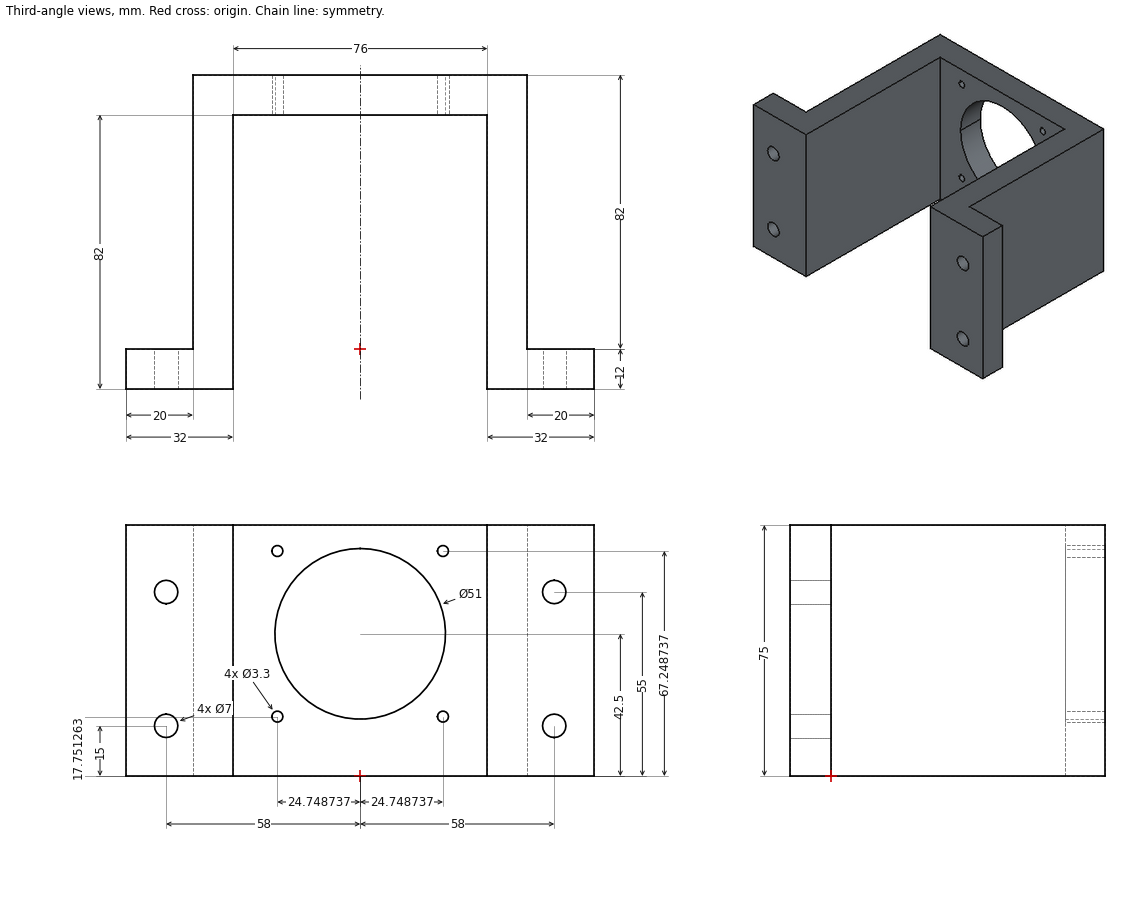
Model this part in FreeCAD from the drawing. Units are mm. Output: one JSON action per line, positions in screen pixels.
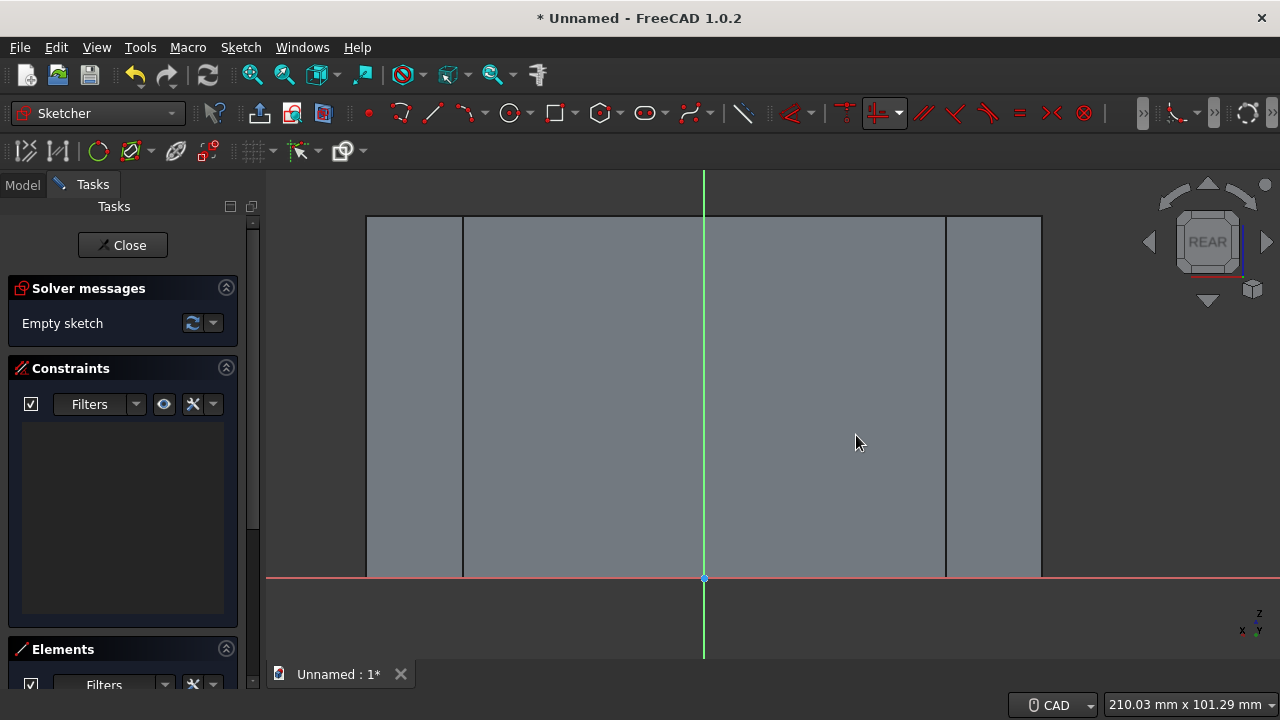
{"action": "left_click", "coordinate": [510, 114]}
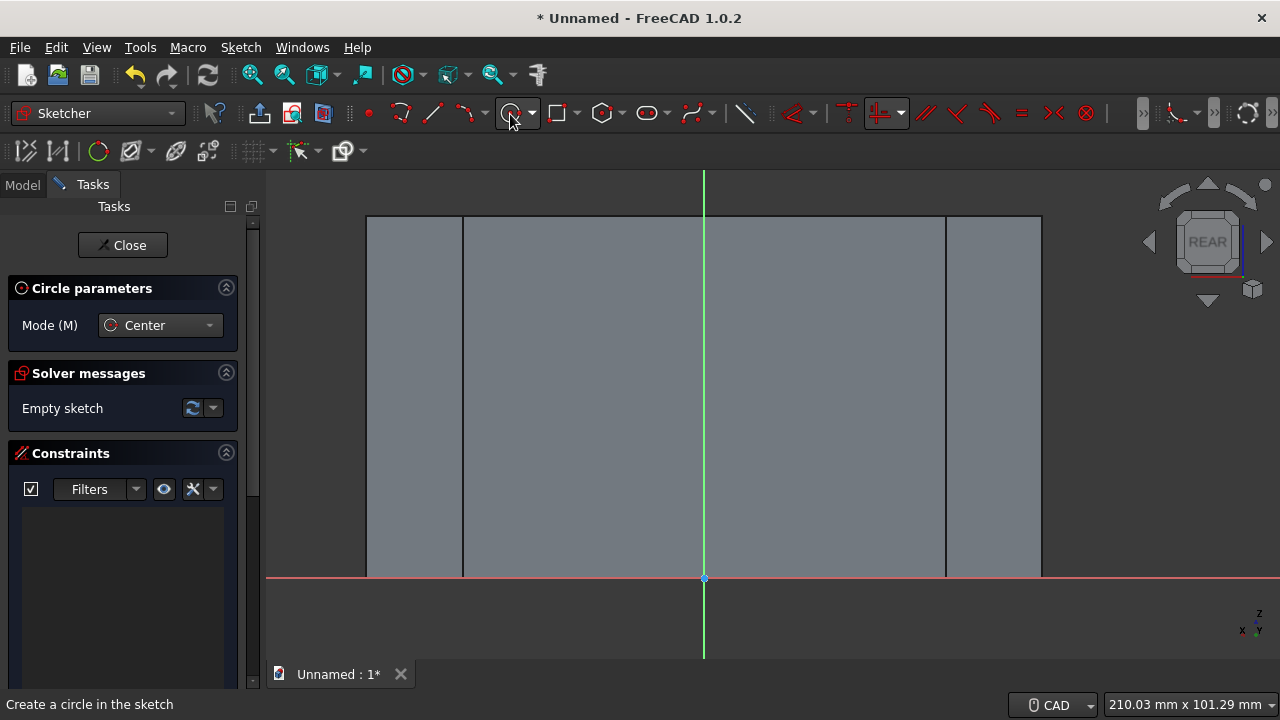
{"action": "left_click", "coordinate": [704, 373]}
{"action": "mouse_move", "coordinate": [791, 286]}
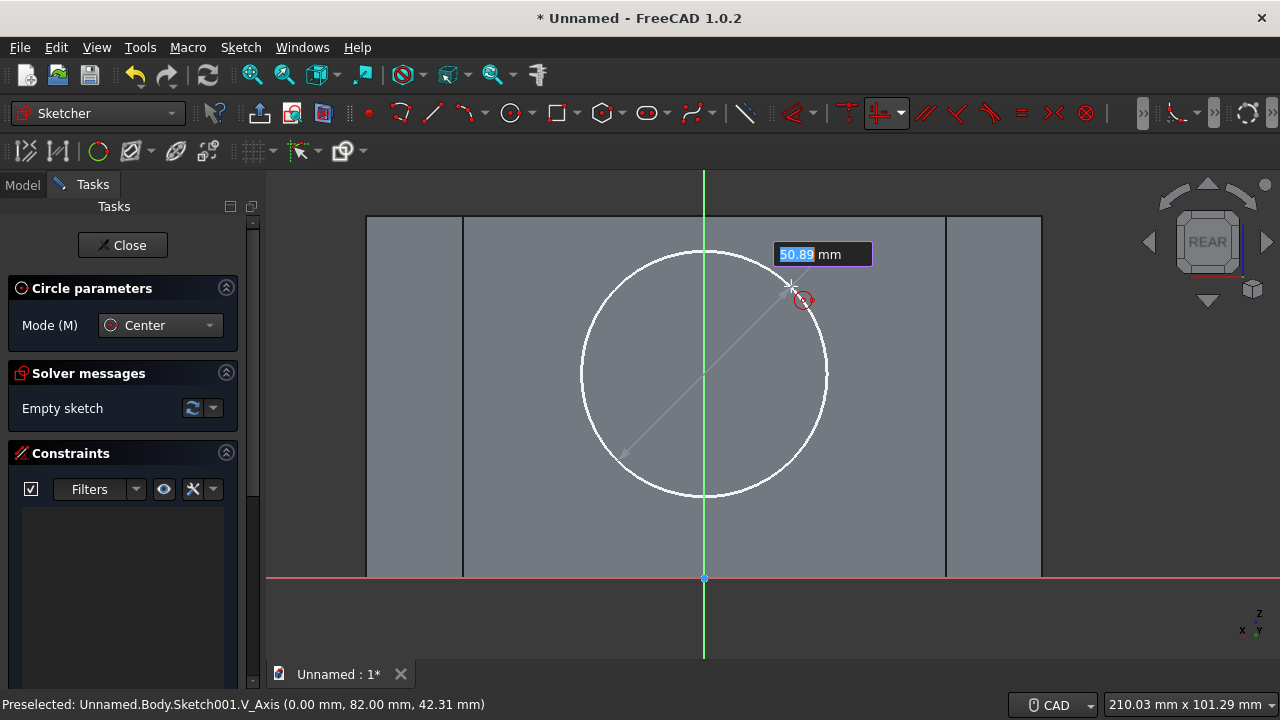
{"action": "type", "text": "51"}
{"action": "key", "text": "Return"}
{"action": "key", "text": "Escape"}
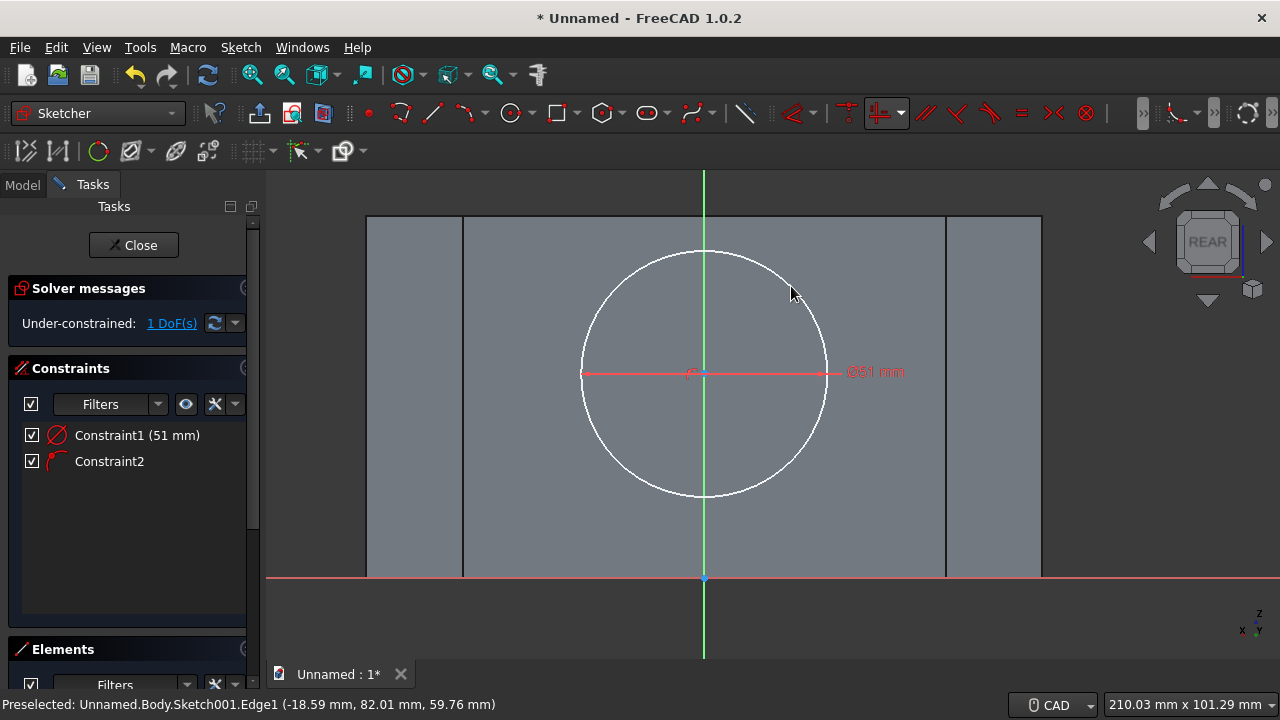
{"action": "left_click", "coordinate": [792, 114]}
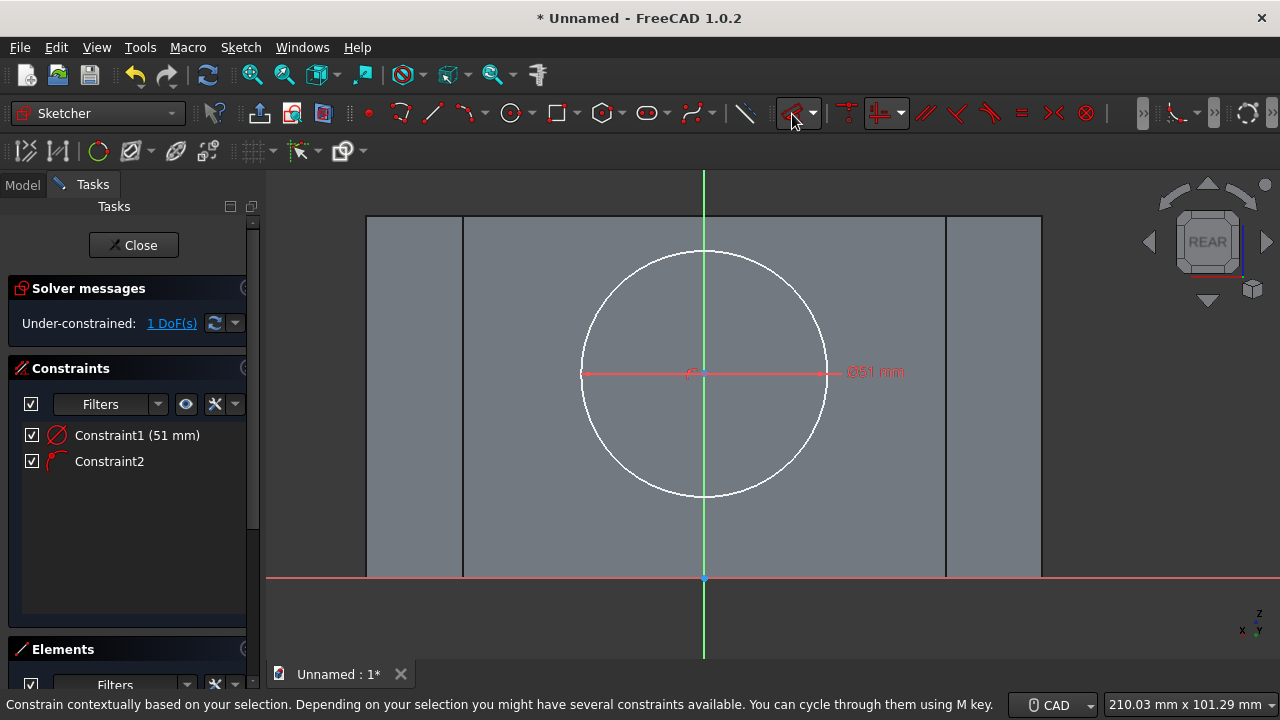
{"action": "left_click", "coordinate": [704, 374]}
{"action": "left_click", "coordinate": [738, 476]}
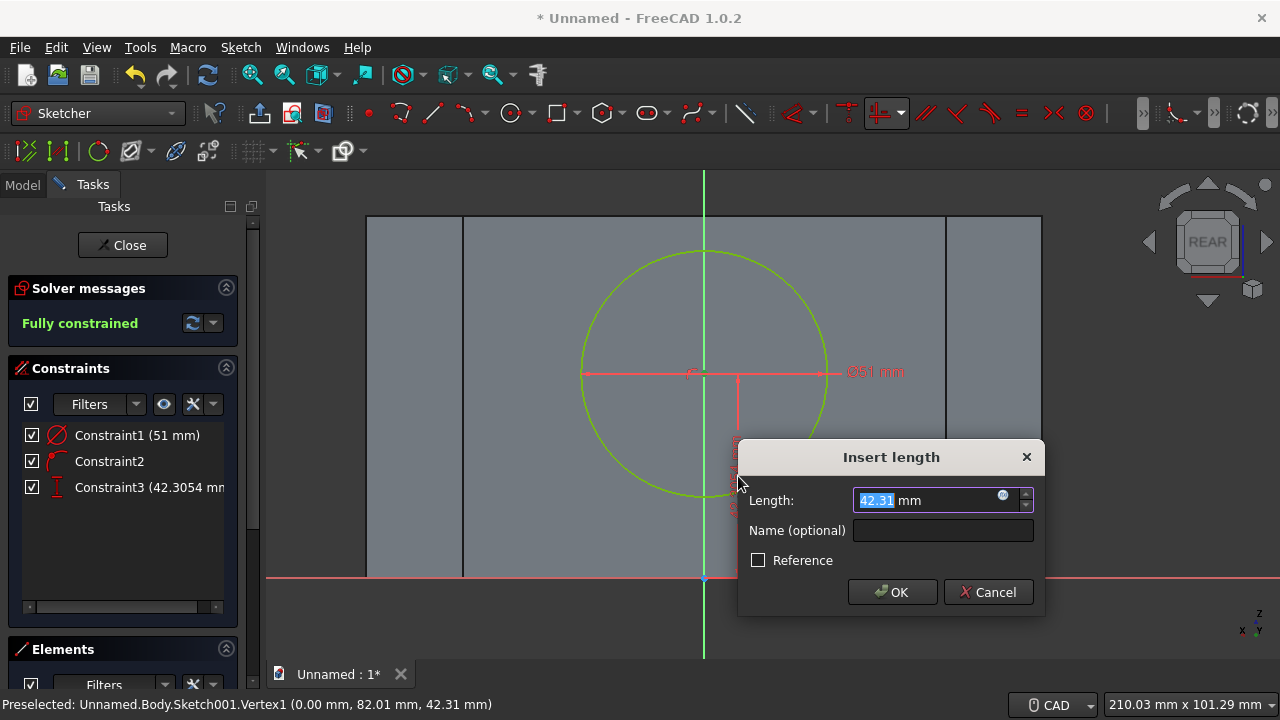
{"action": "type", "text": "42.5"}
{"action": "key", "text": "Return"}
{"action": "key", "text": "Escape"}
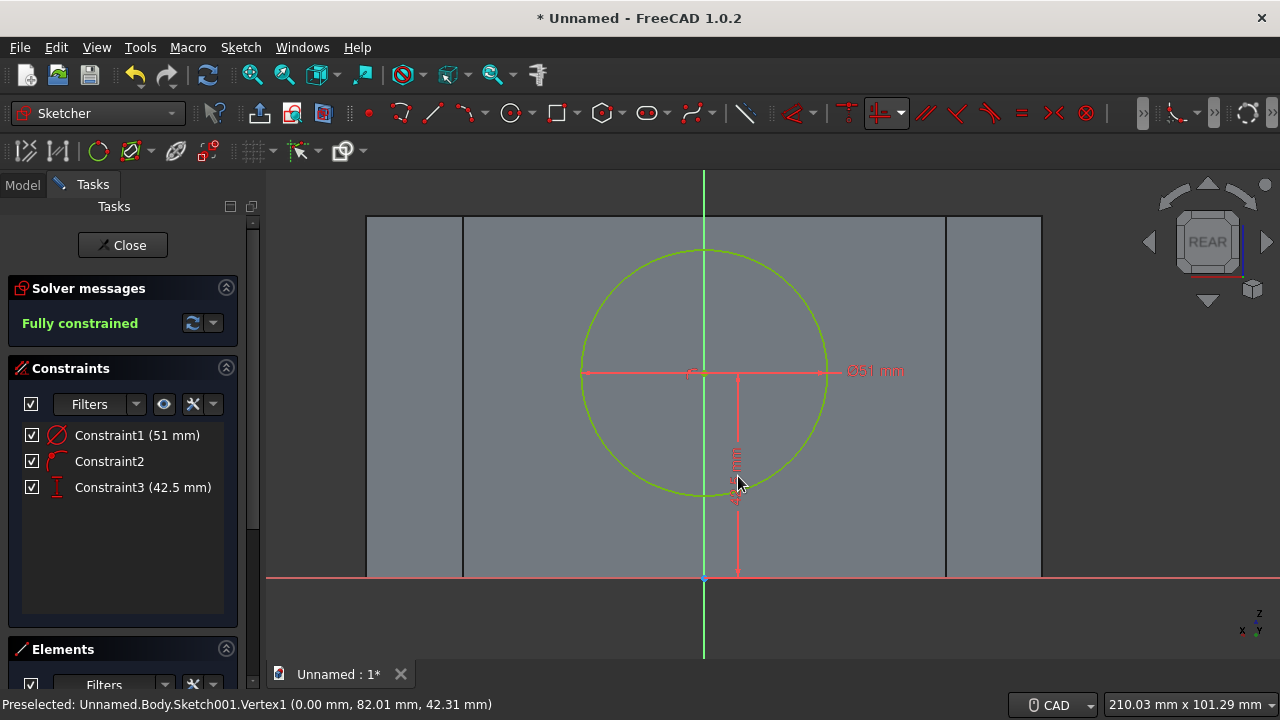
{"action": "left_click", "coordinate": [123, 245]}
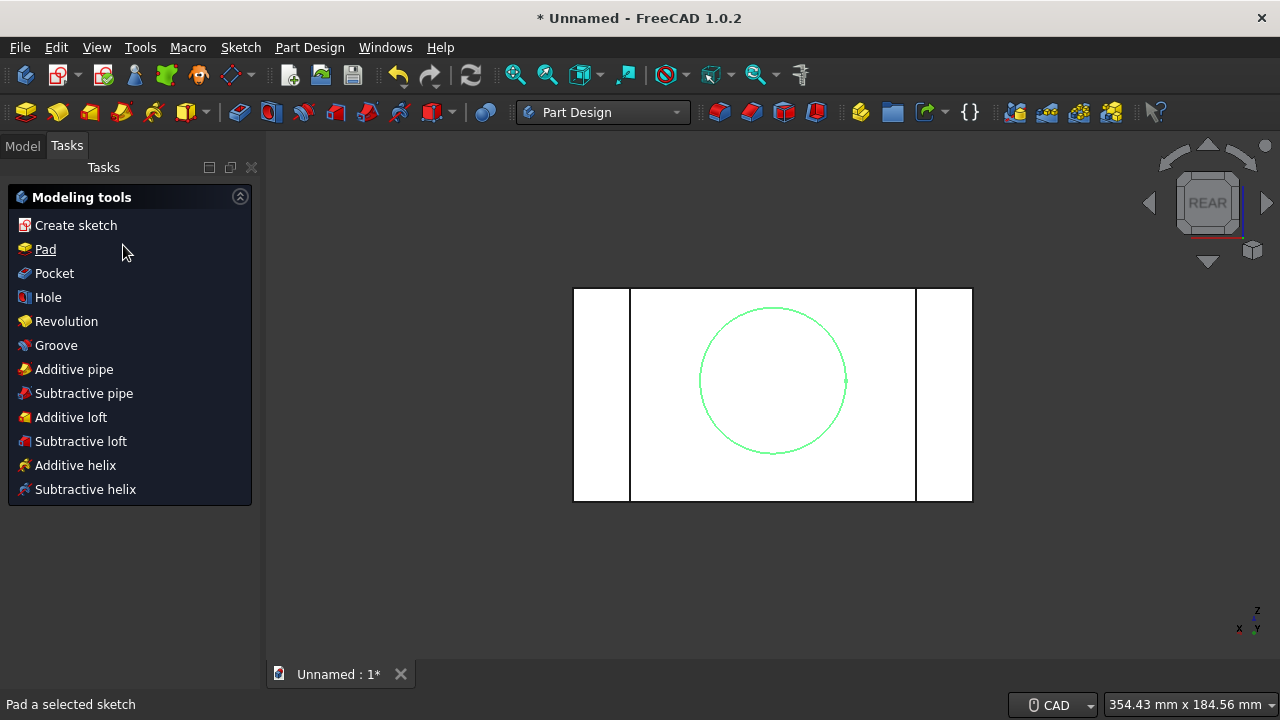
{"action": "left_click", "coordinate": [240, 112]}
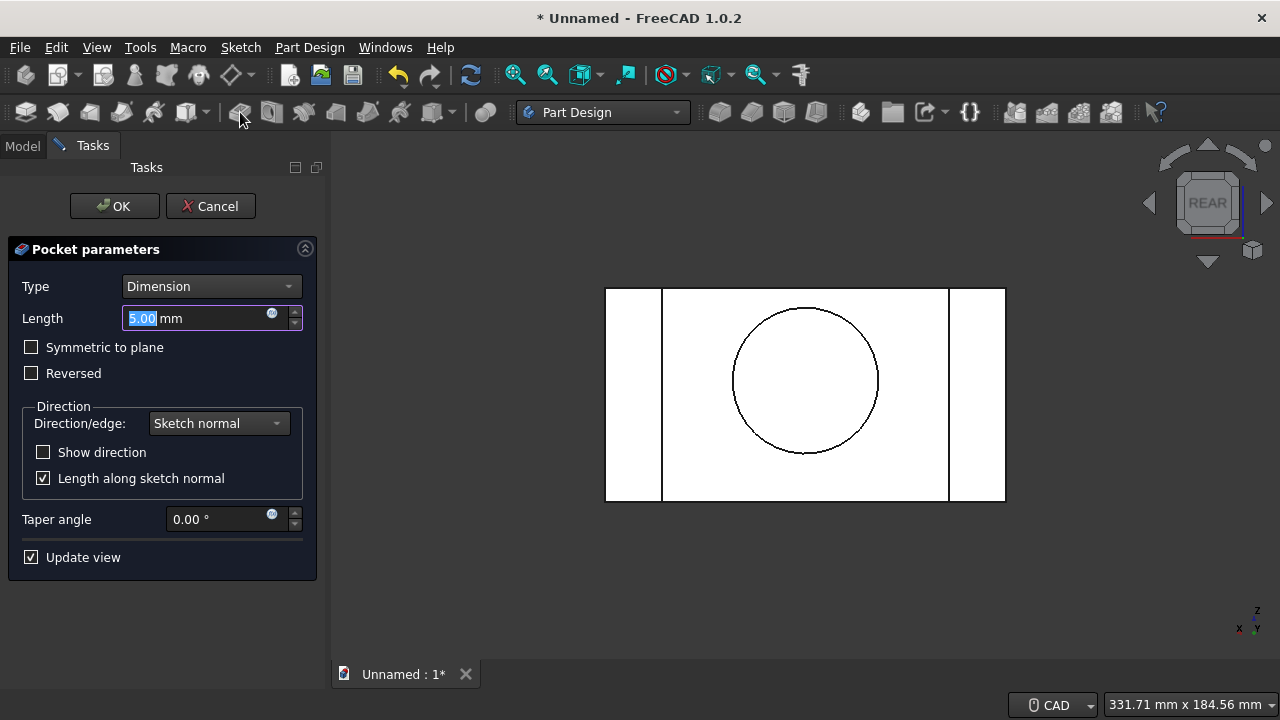
{"action": "left_click", "coordinate": [212, 286]}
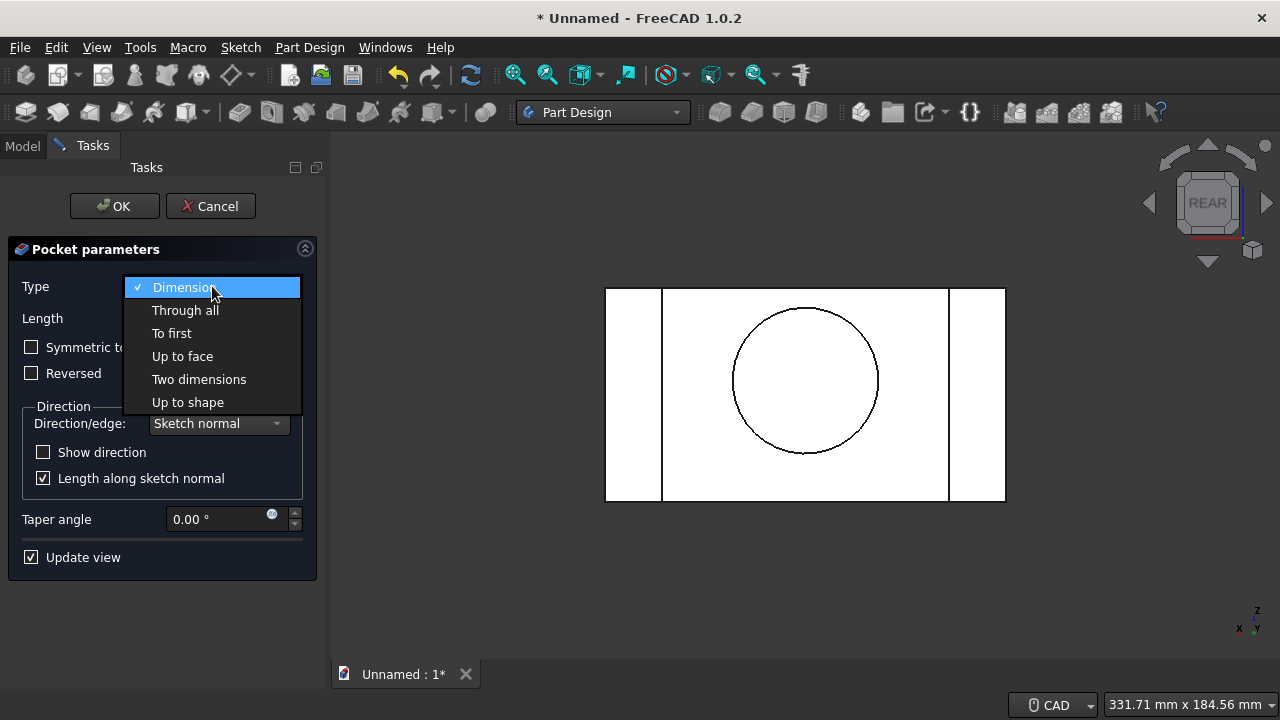
{"action": "left_click", "coordinate": [212, 310]}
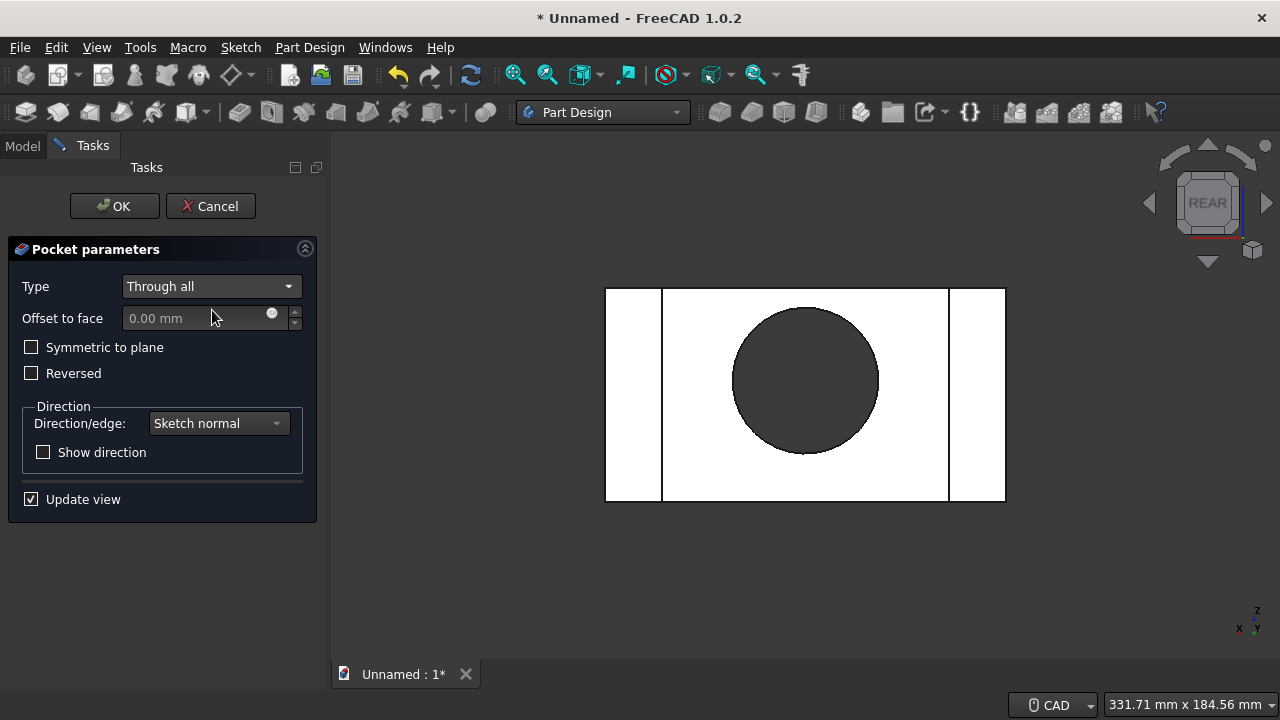
{"action": "left_click", "coordinate": [115, 206]}